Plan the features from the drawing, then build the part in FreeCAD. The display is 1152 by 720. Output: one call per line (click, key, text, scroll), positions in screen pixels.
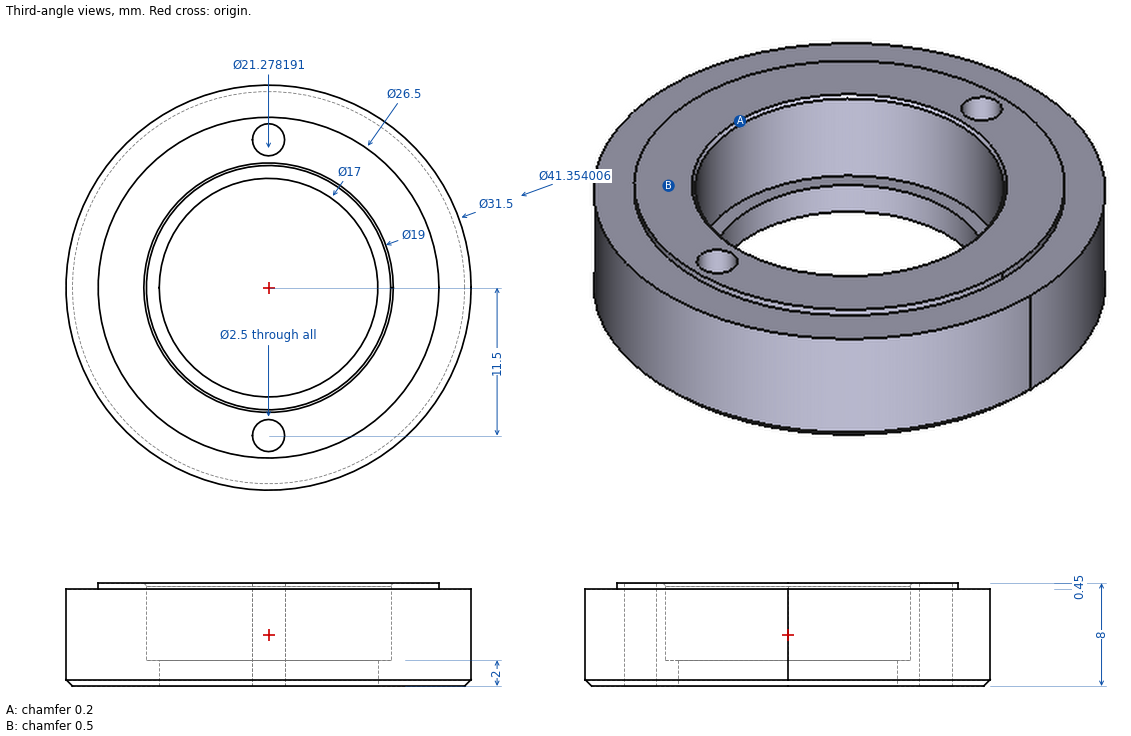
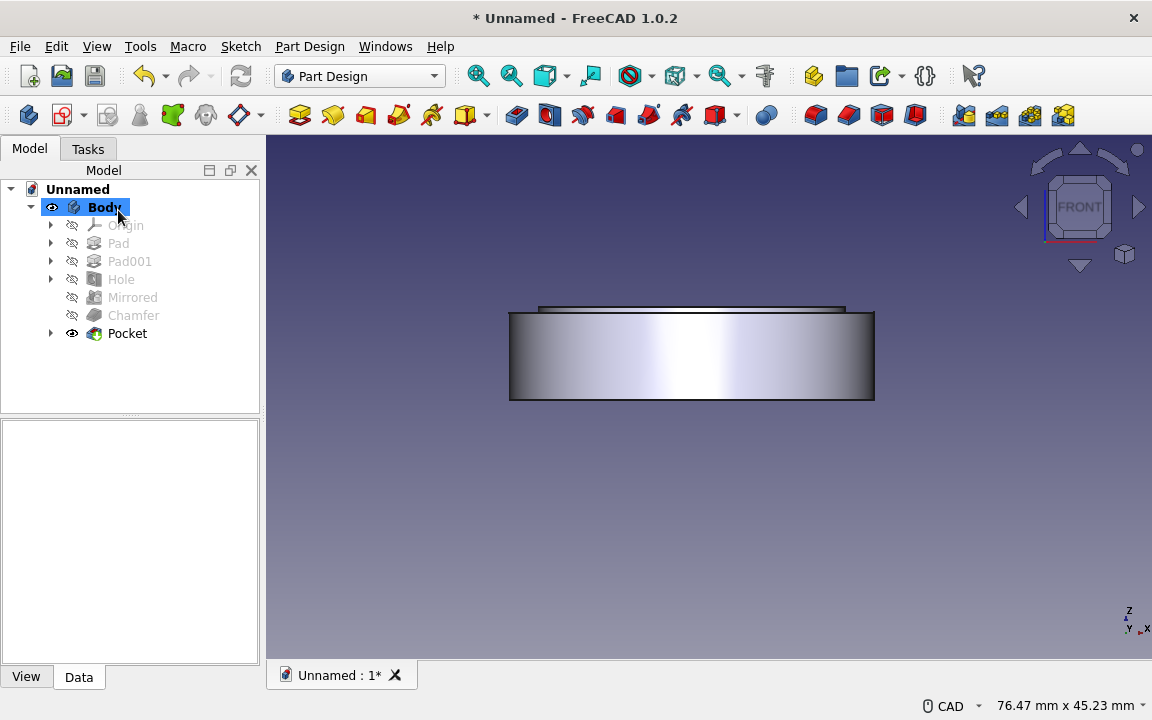
click(479, 76)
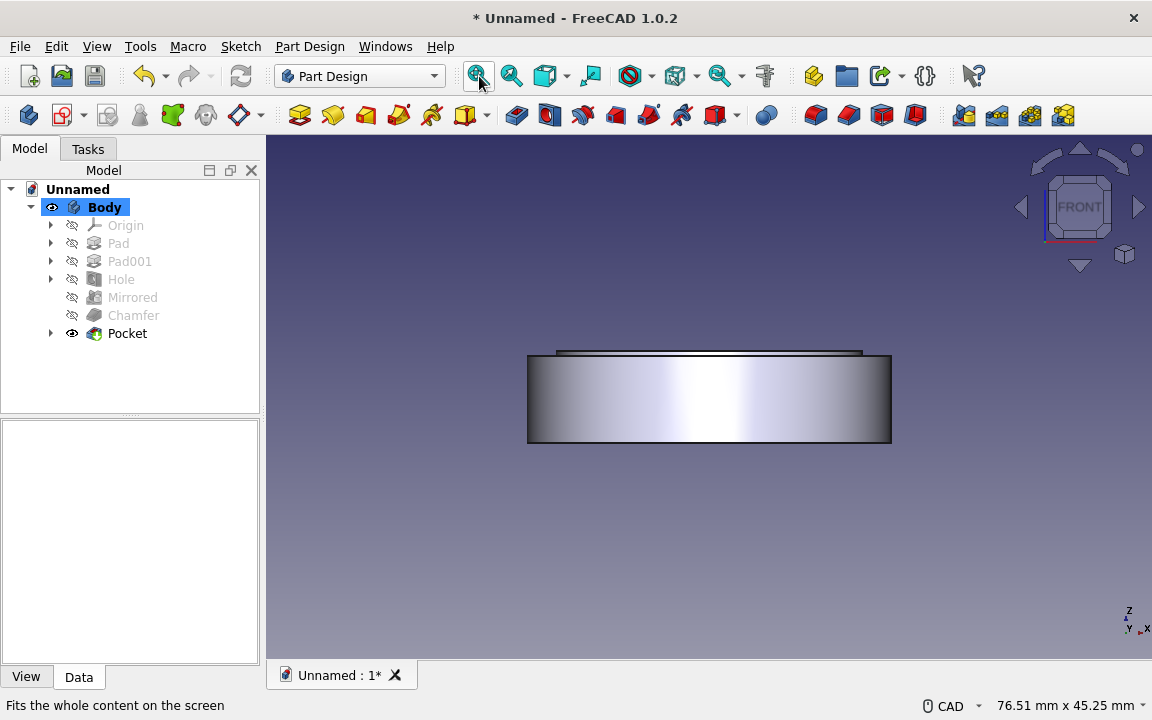
click(653, 442)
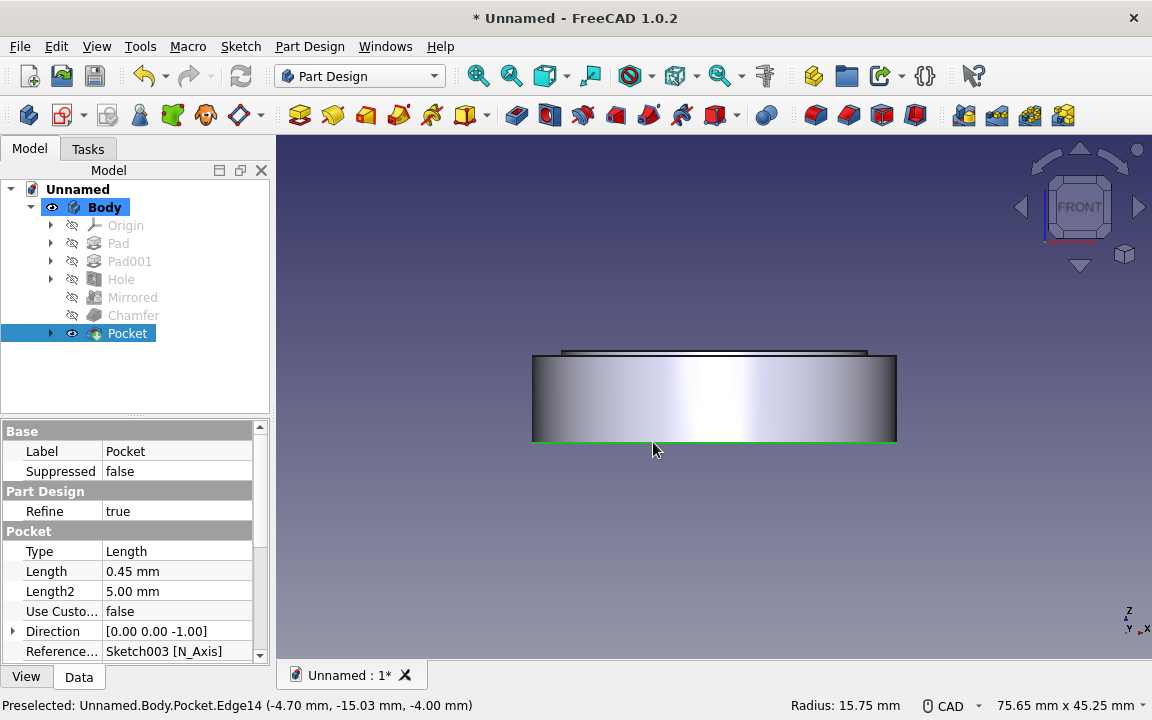
click(849, 116)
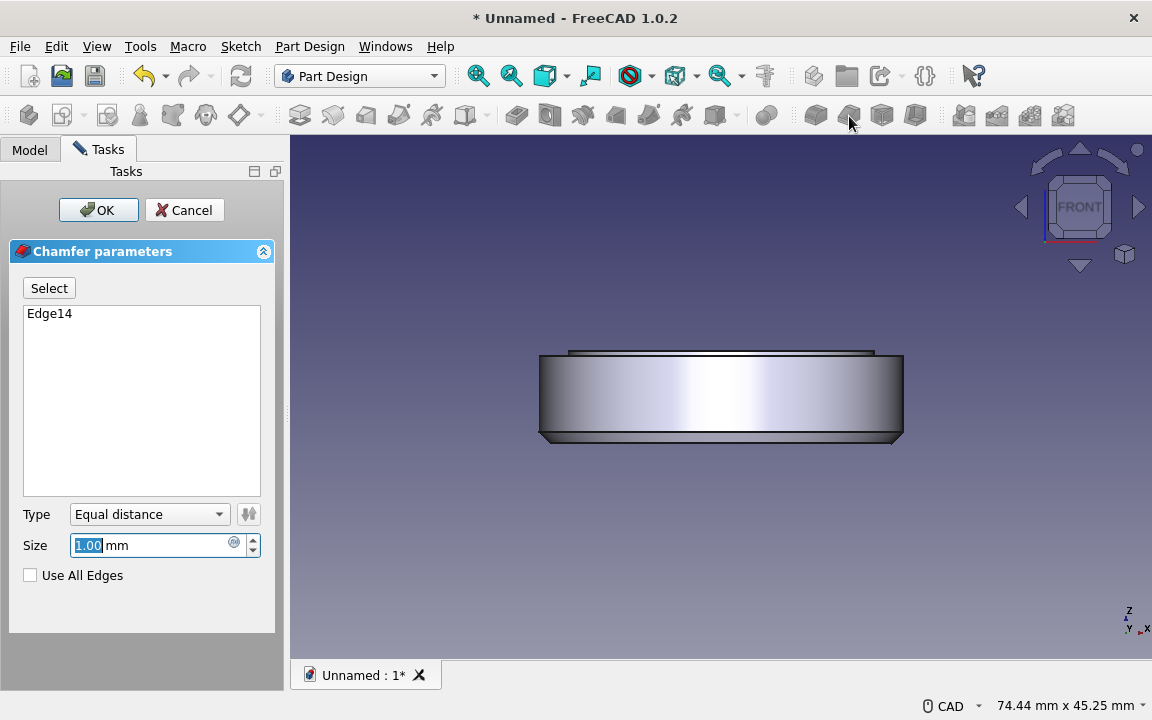
text(0.5)
key(Tab)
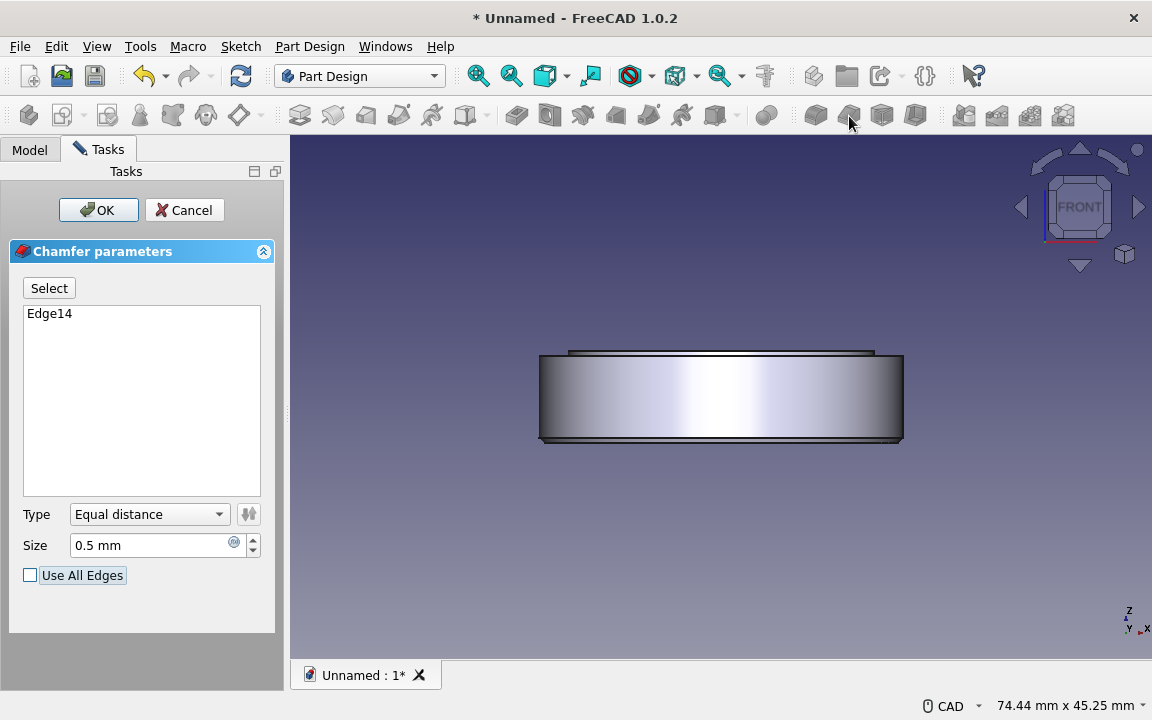
click(99, 210)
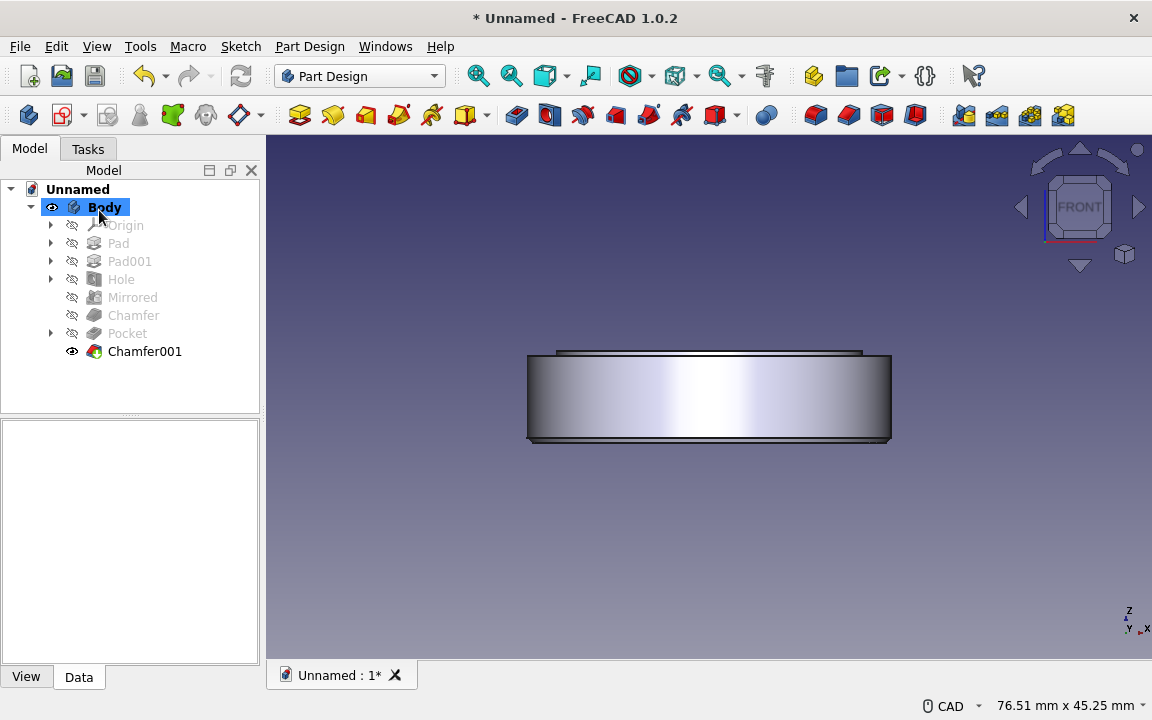
key(0)